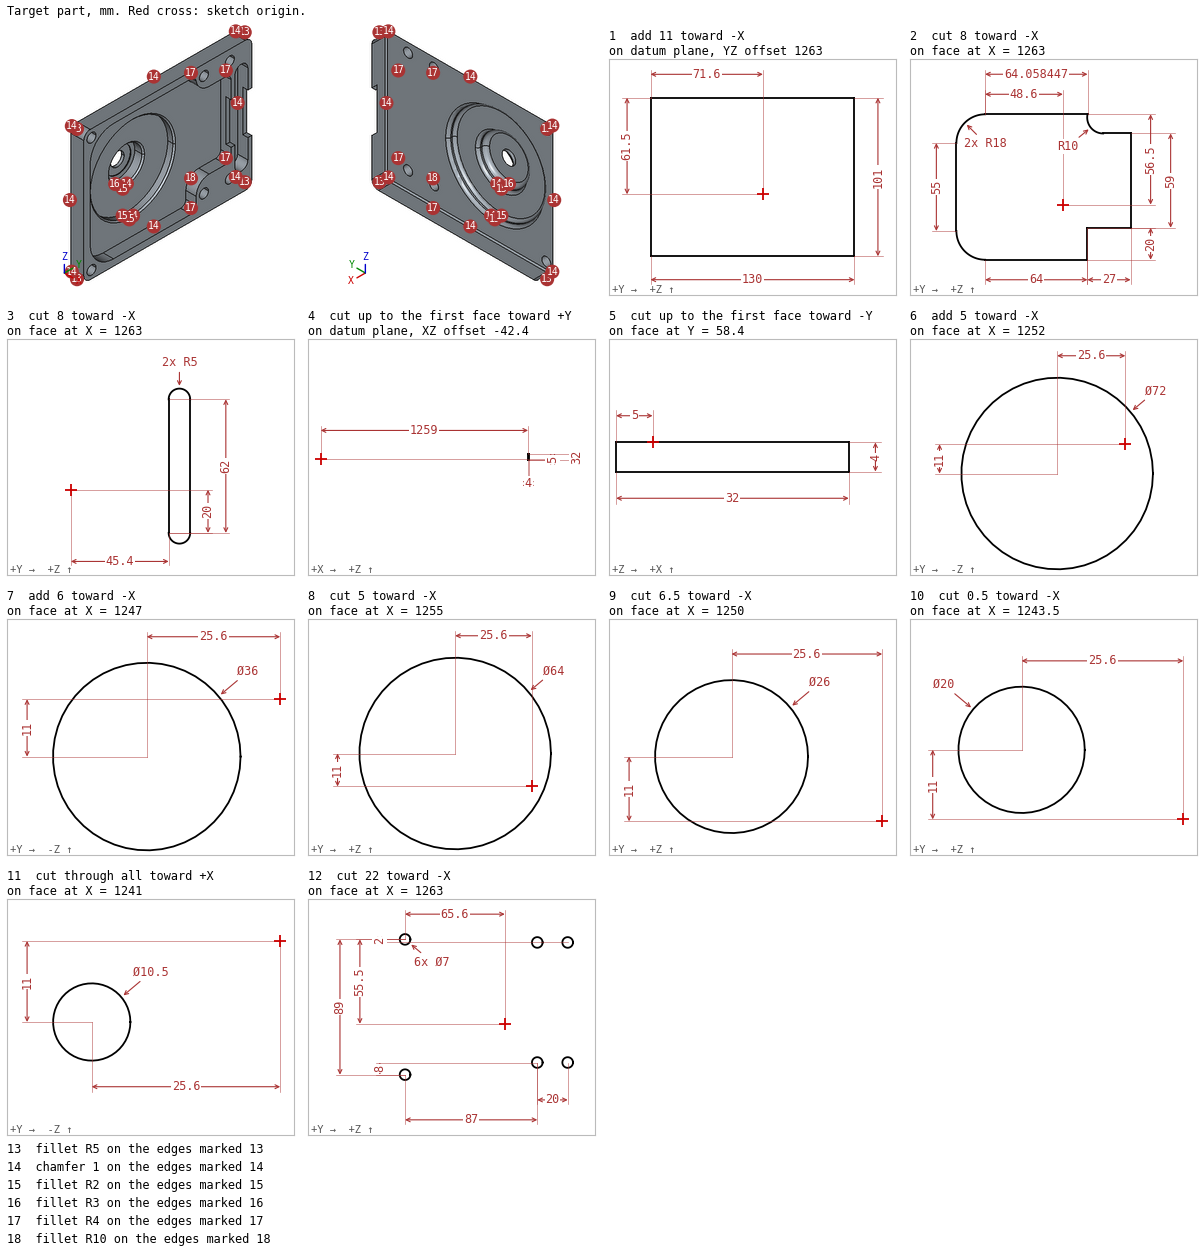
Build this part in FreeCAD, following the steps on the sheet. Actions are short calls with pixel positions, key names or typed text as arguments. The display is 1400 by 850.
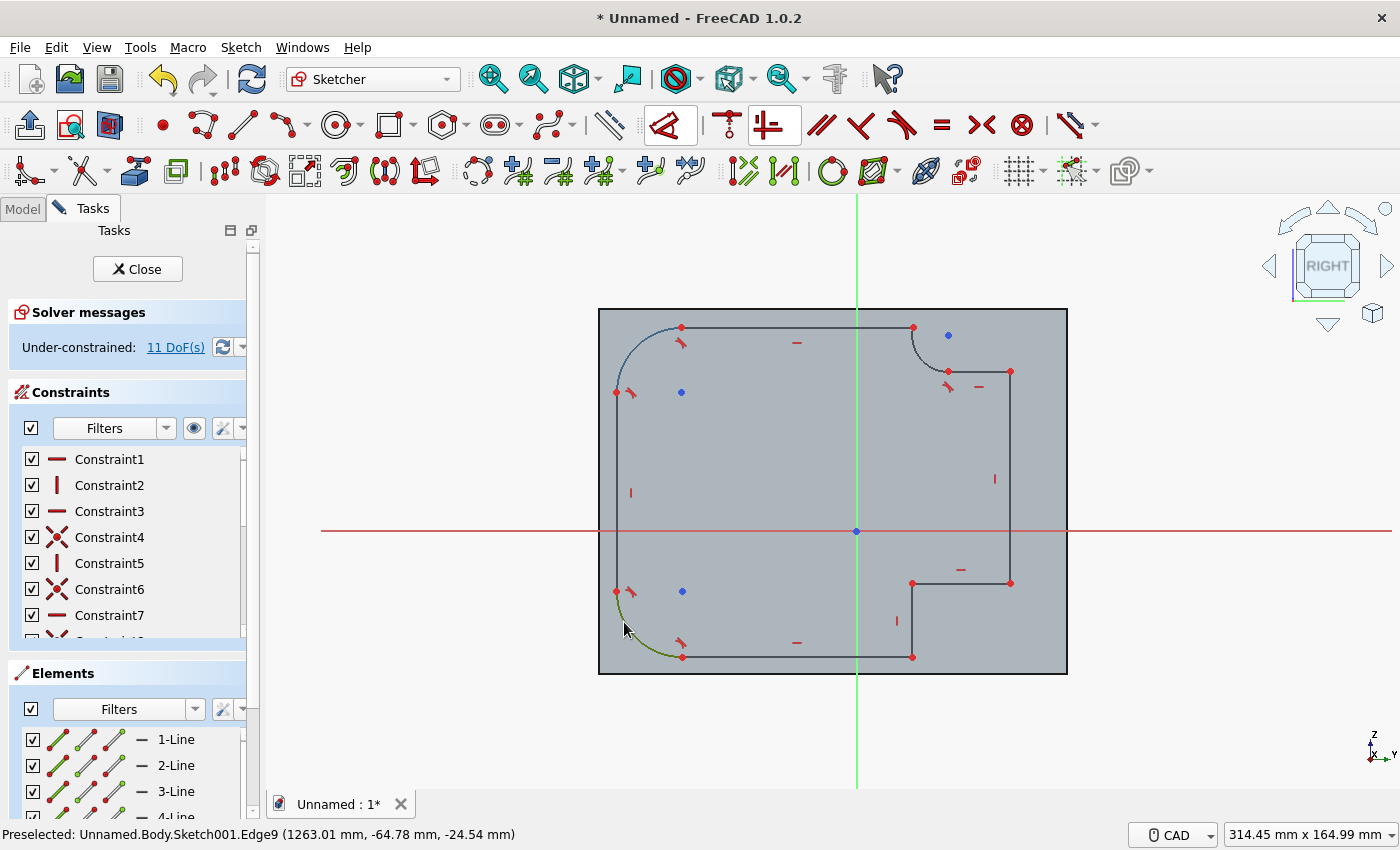
key(e)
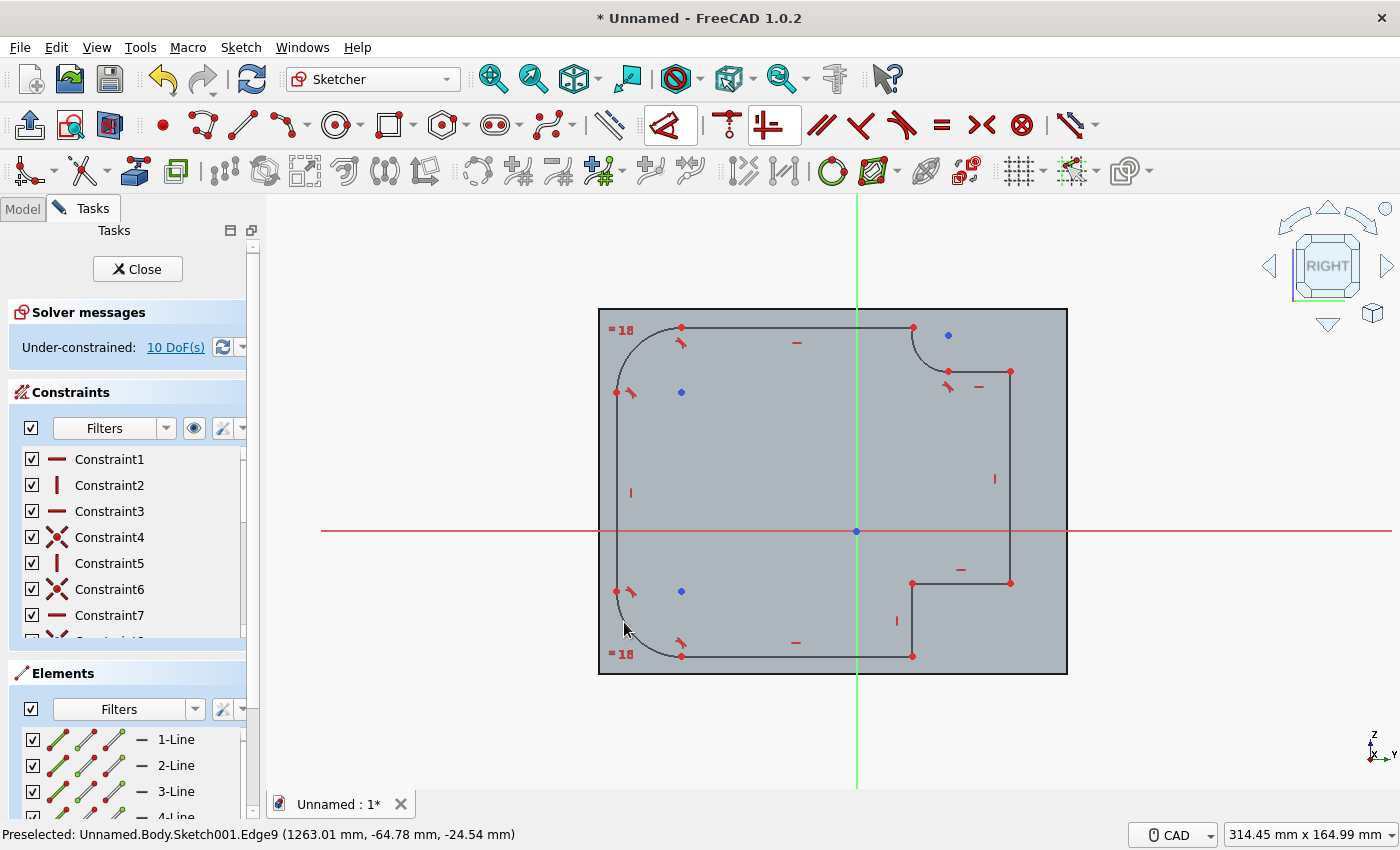
click(652, 335)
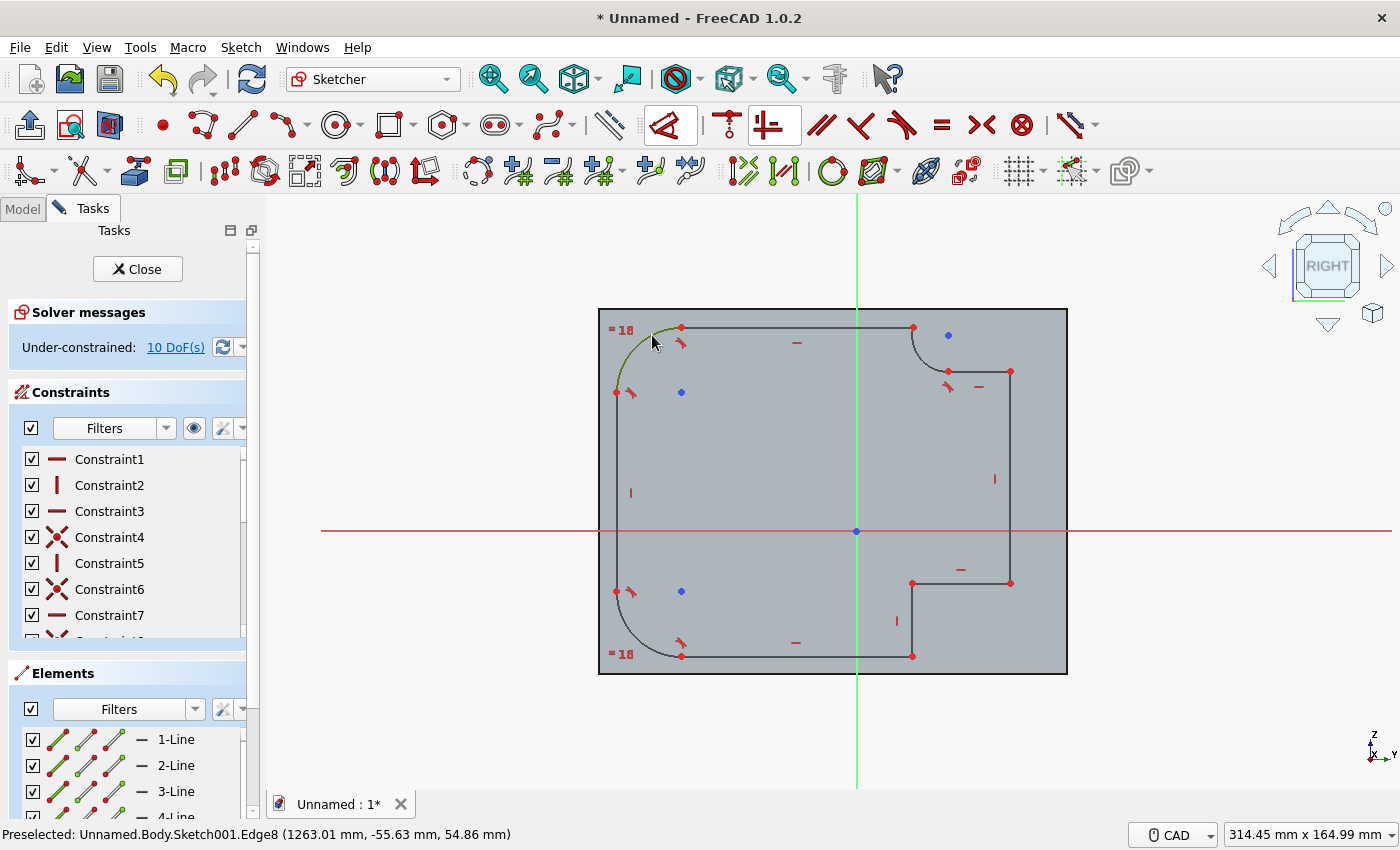
click(692, 126)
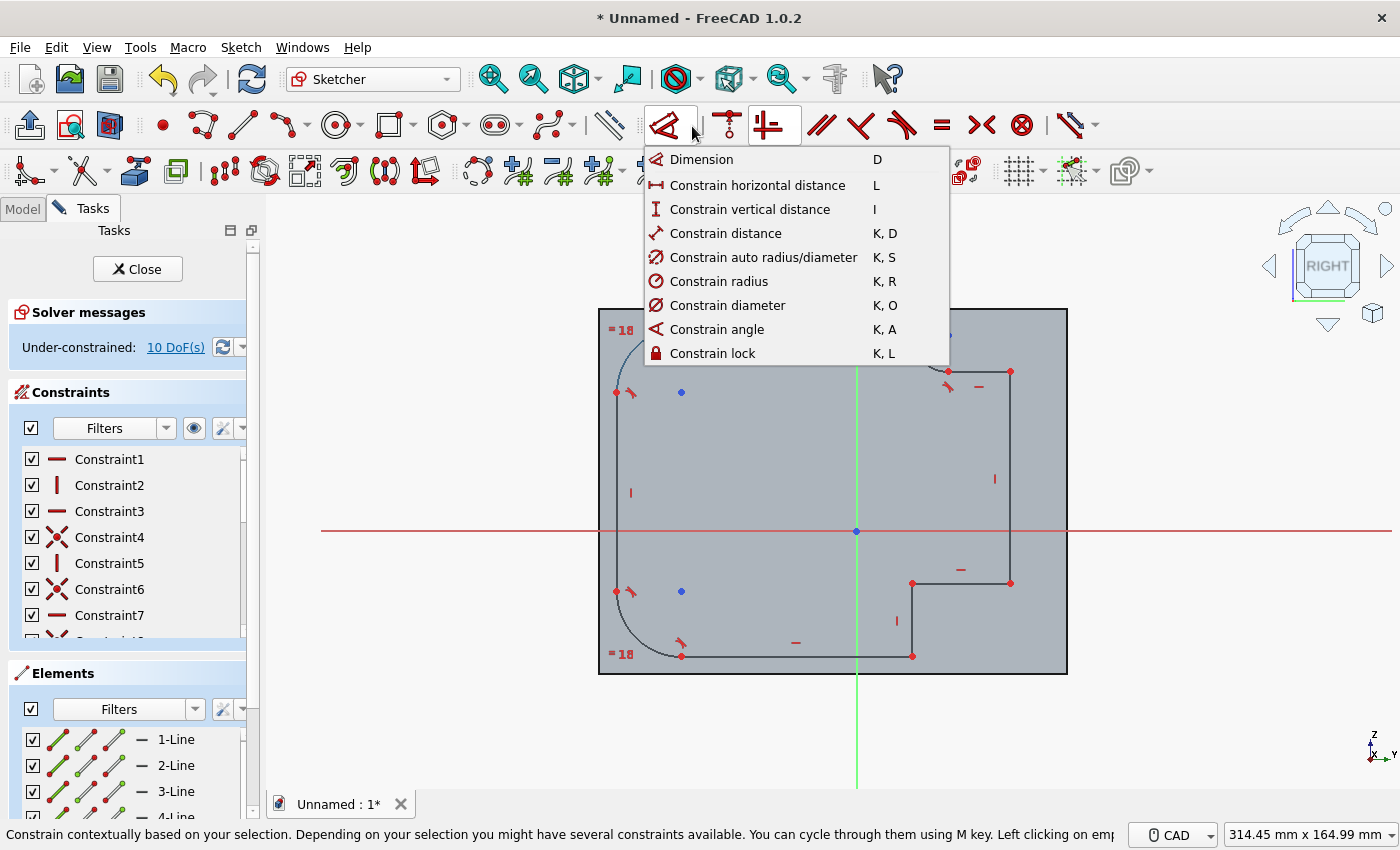
click(797, 281)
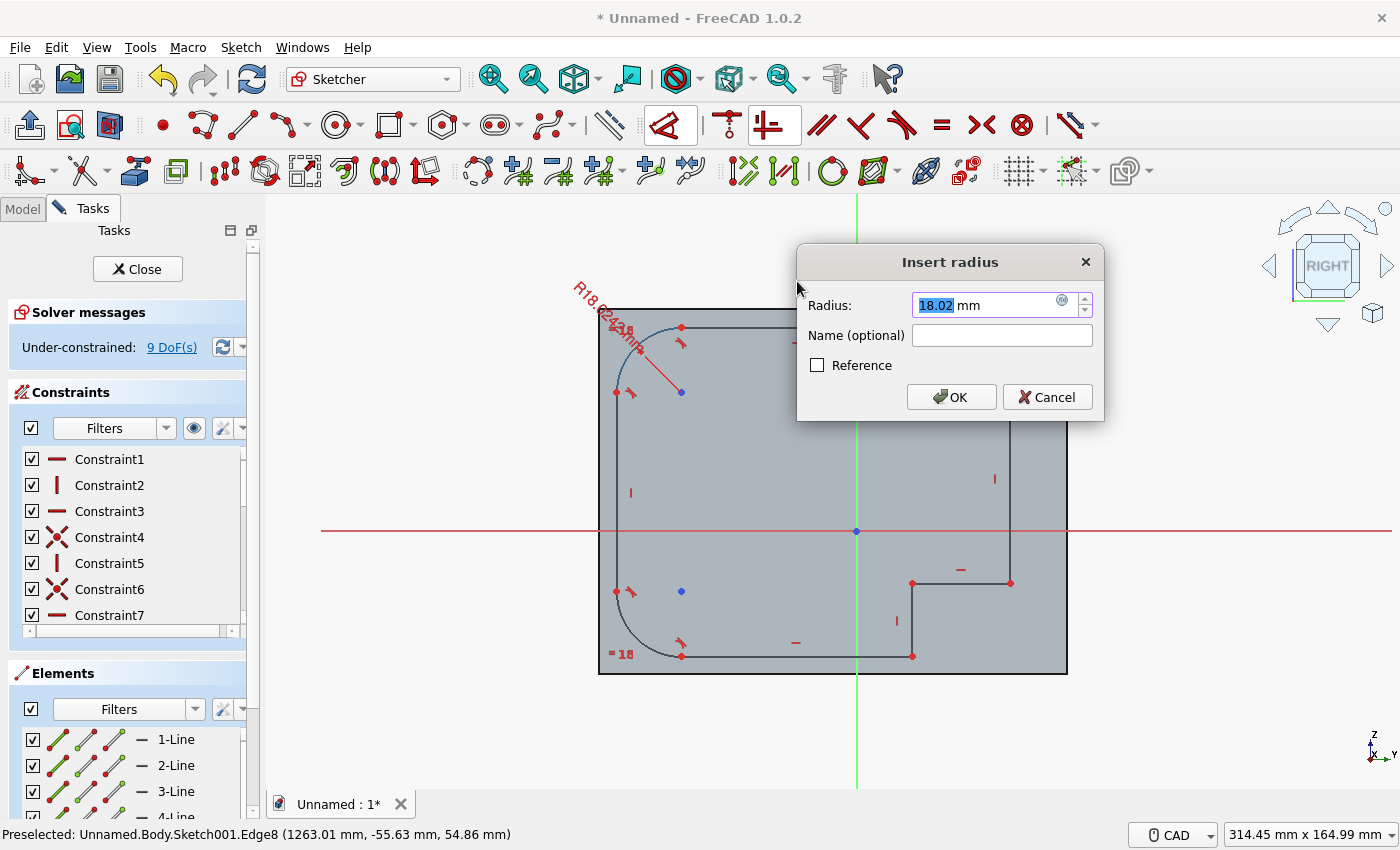
text(18)
key(Return)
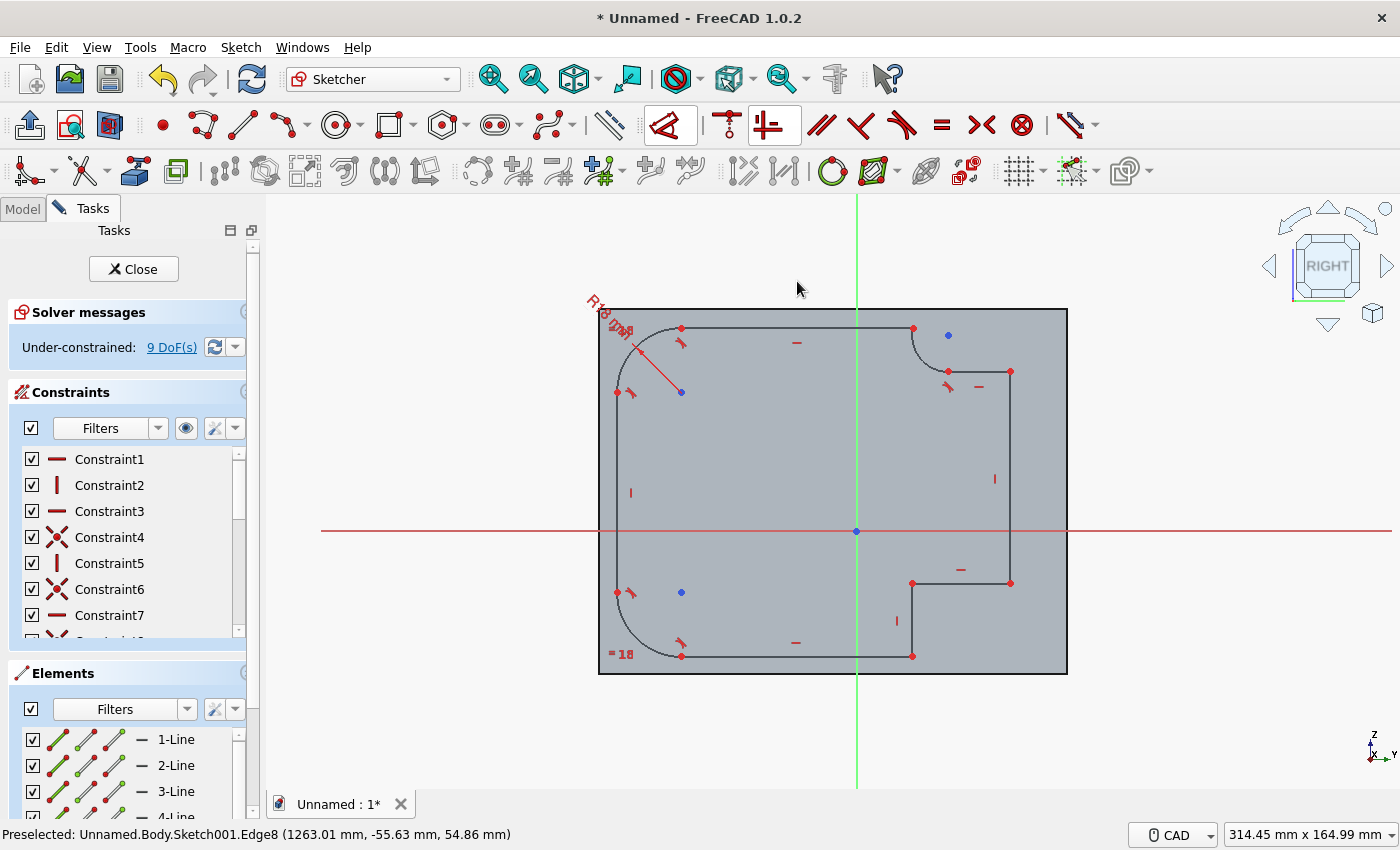
click(914, 347)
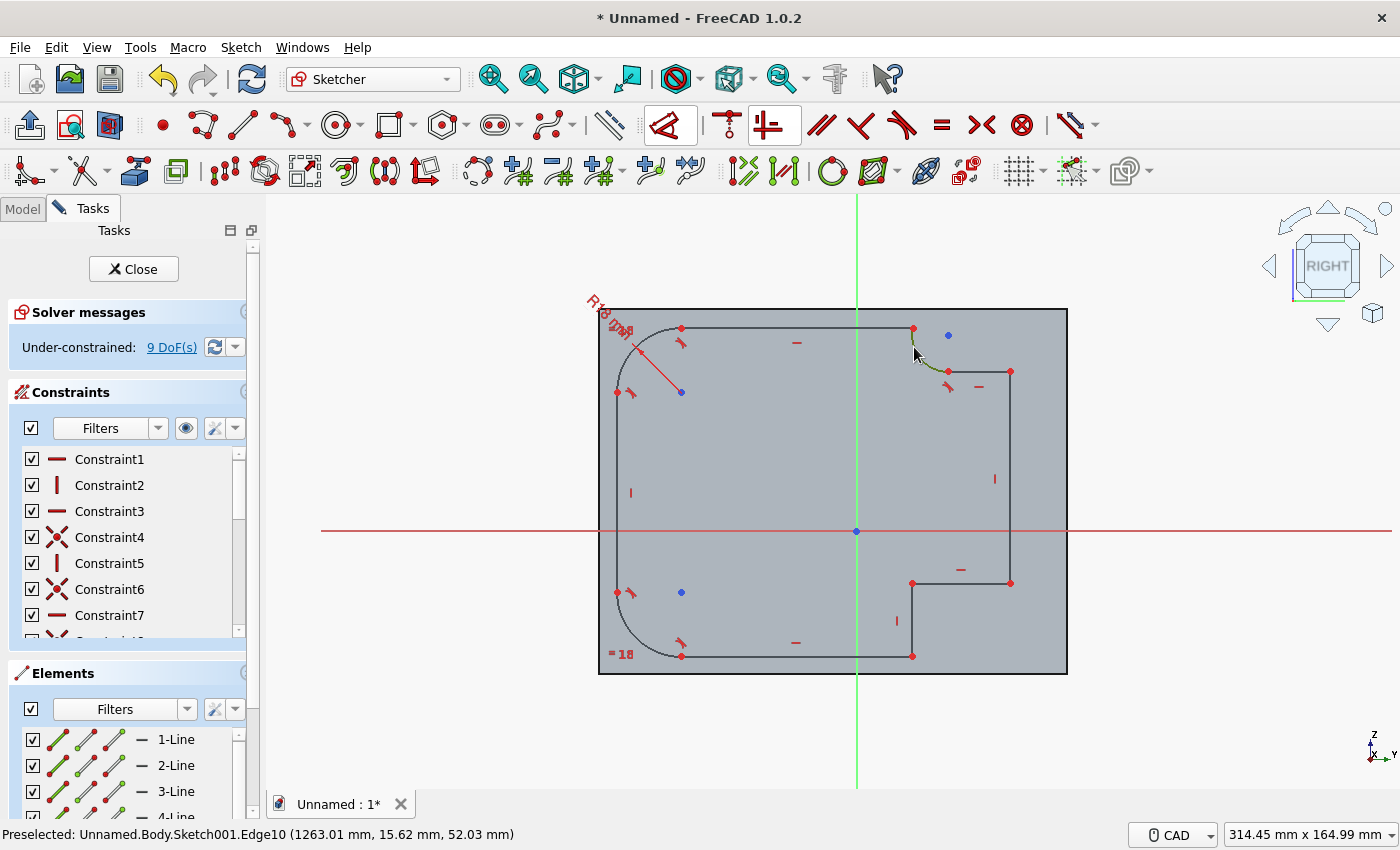
key(k)
key(r)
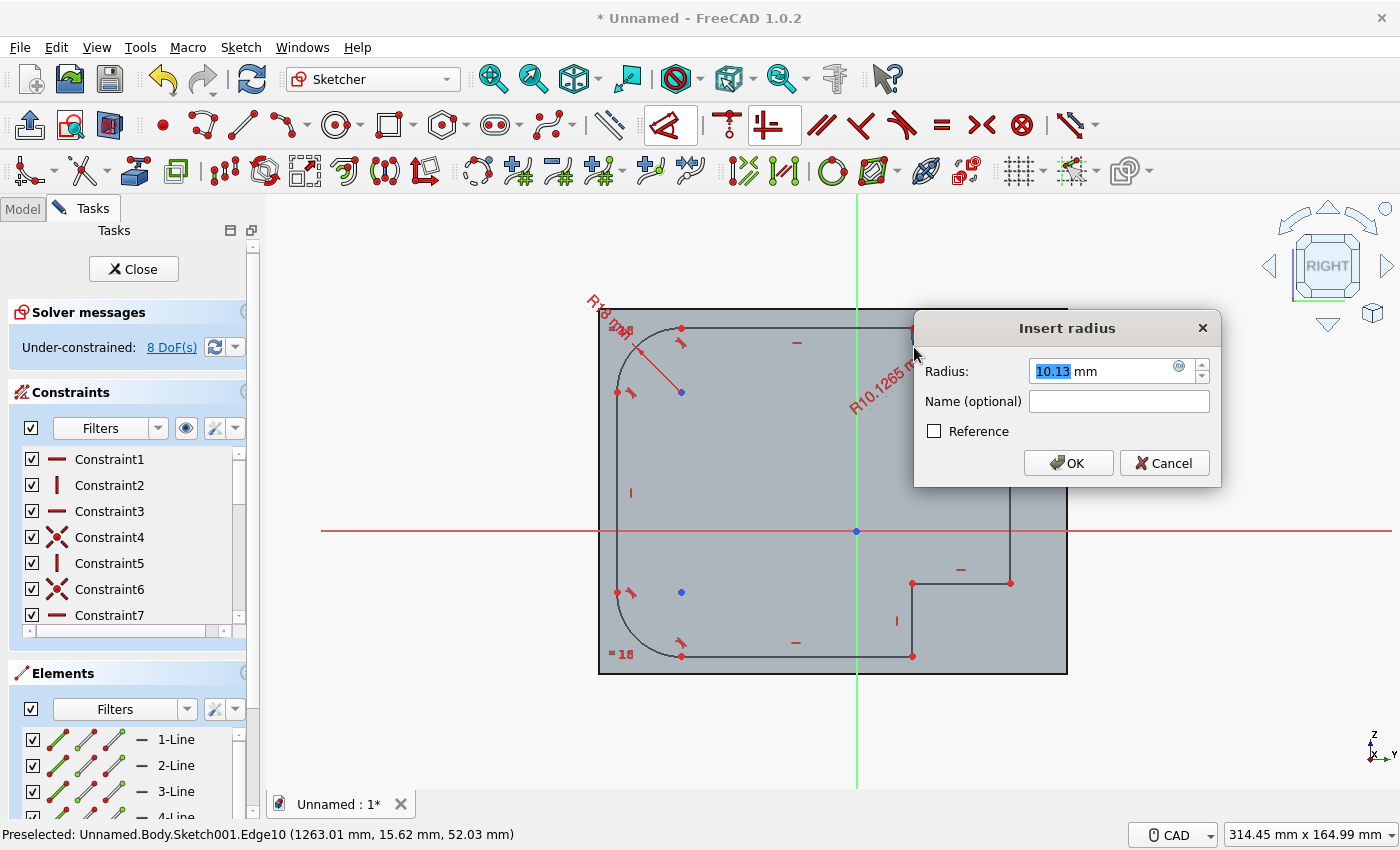
text(10)
key(Return)